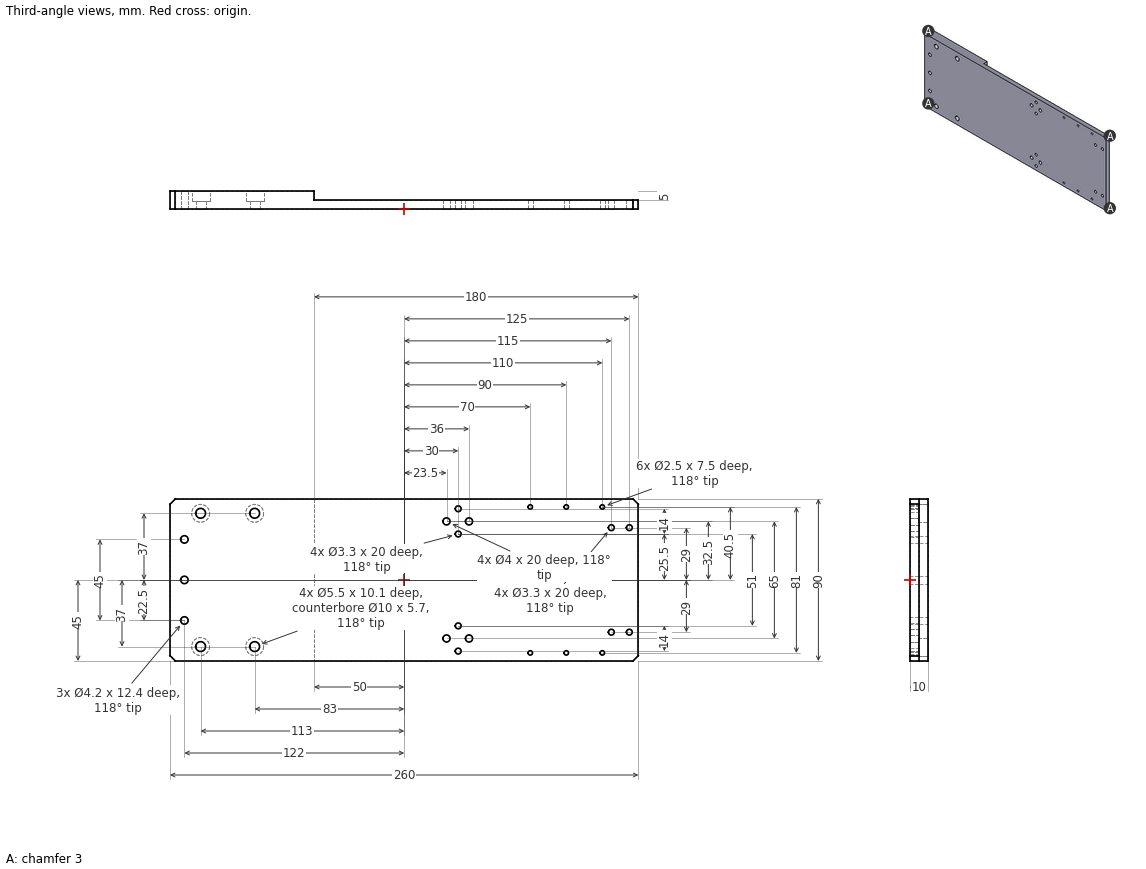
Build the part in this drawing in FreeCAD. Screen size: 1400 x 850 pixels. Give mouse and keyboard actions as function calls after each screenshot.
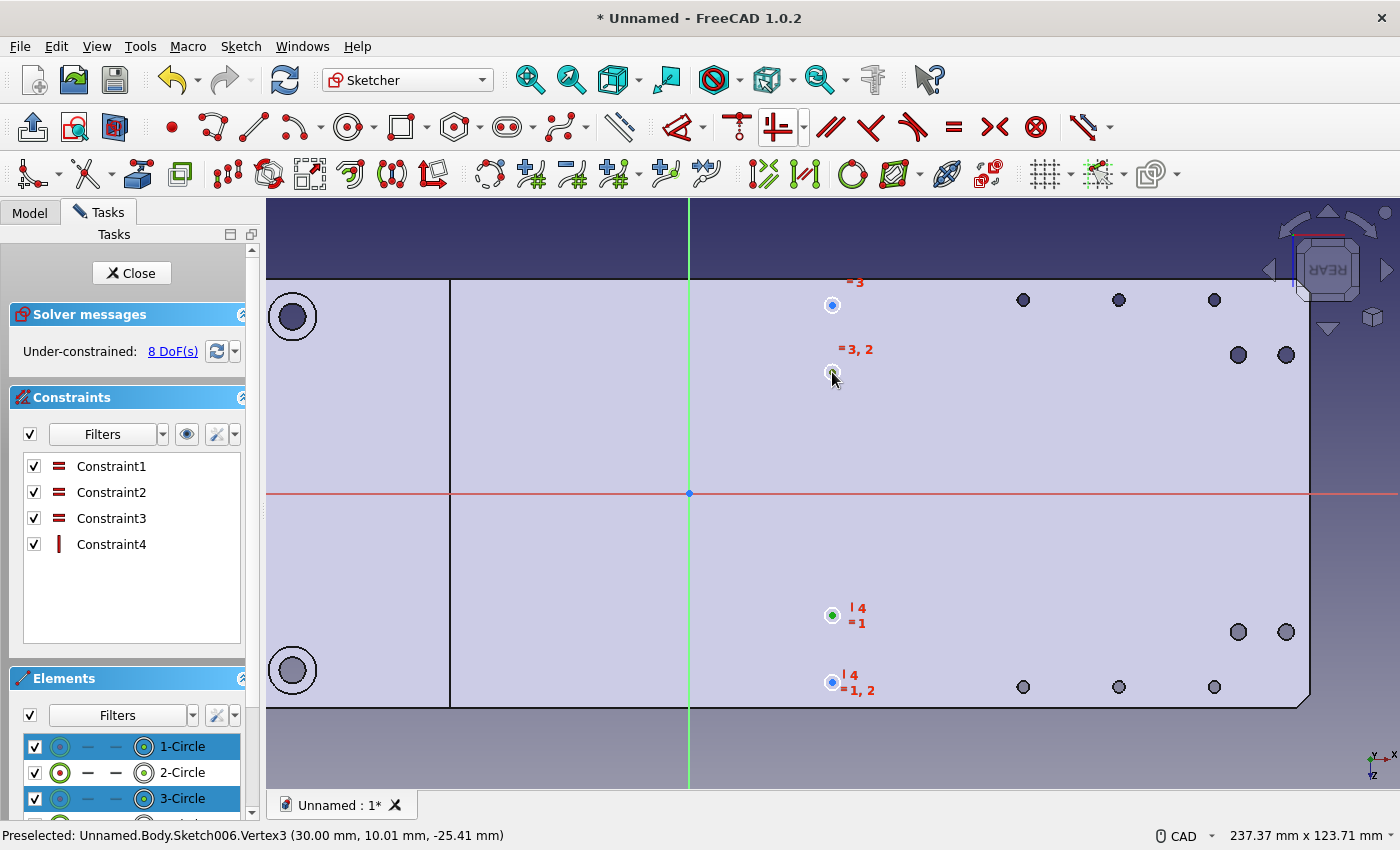
click(804, 128)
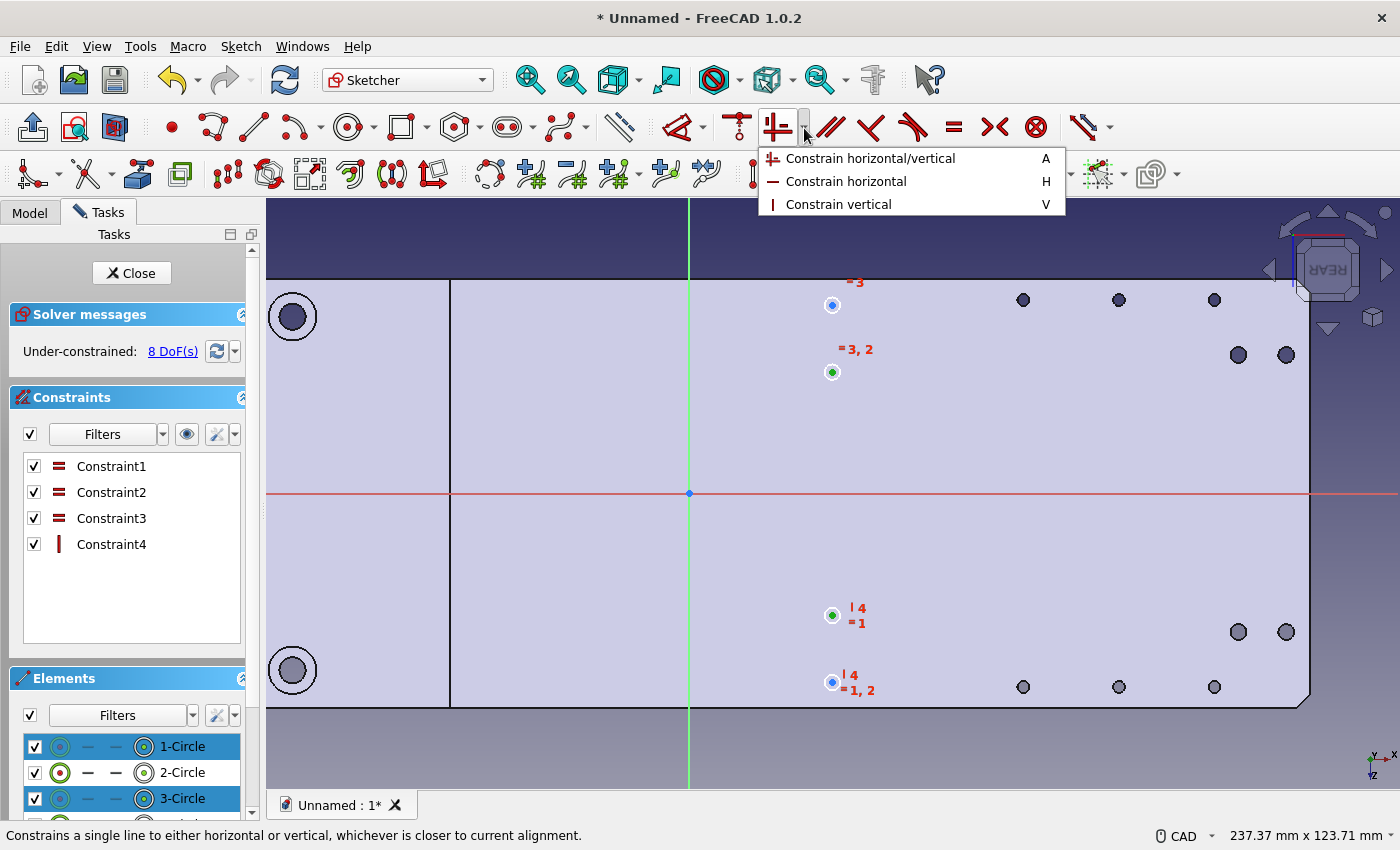
click(912, 204)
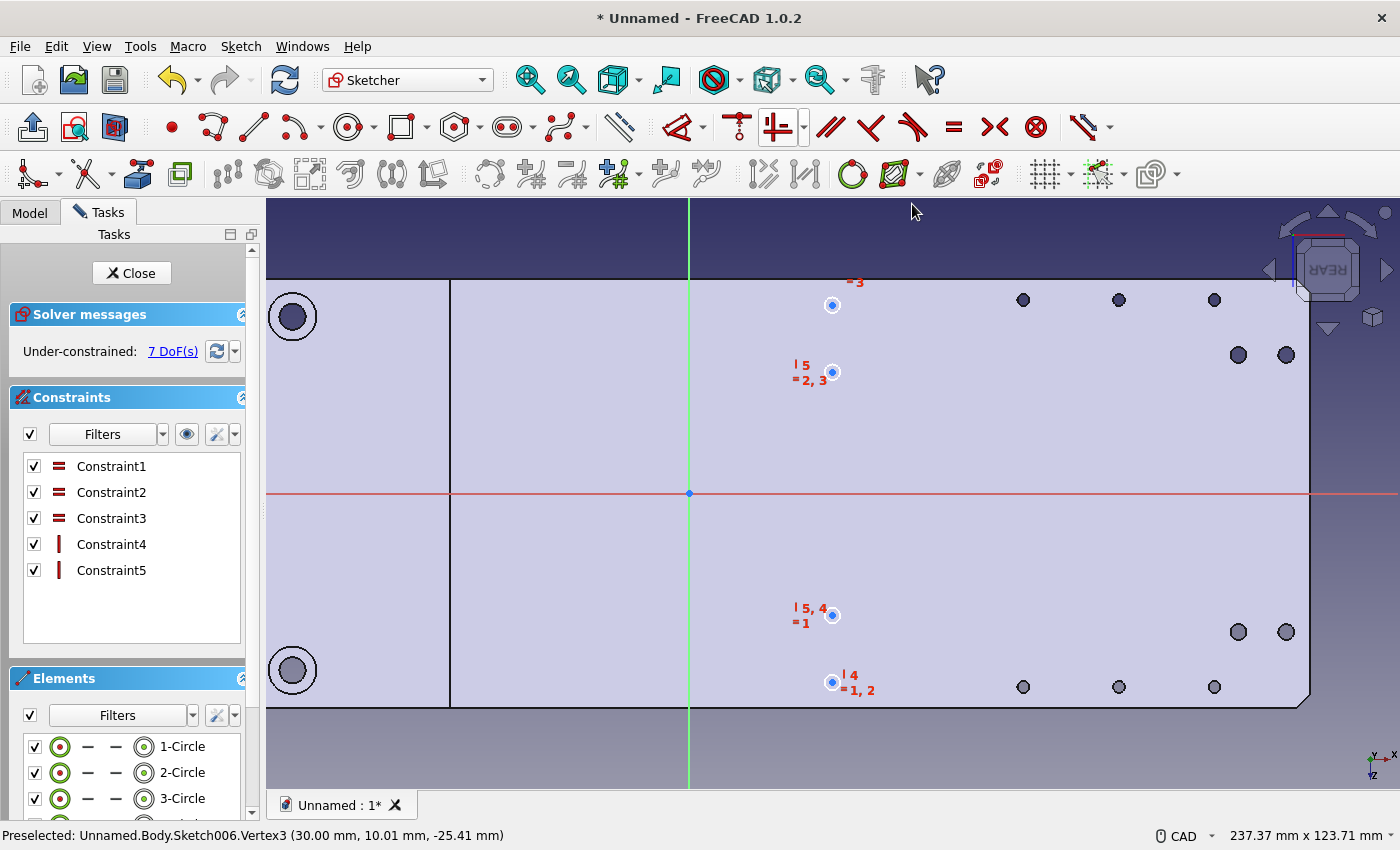
click(832, 372)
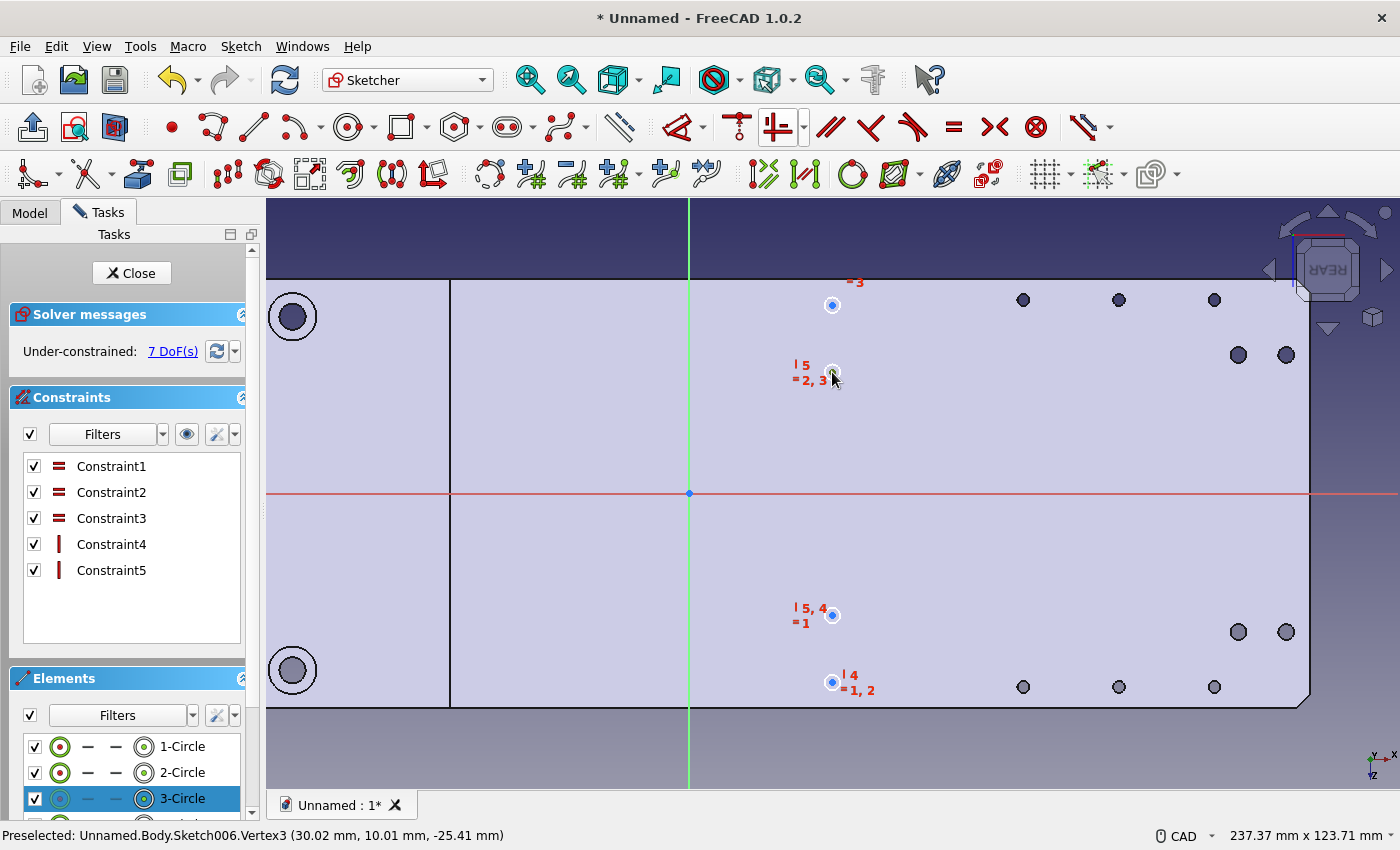
click(832, 305)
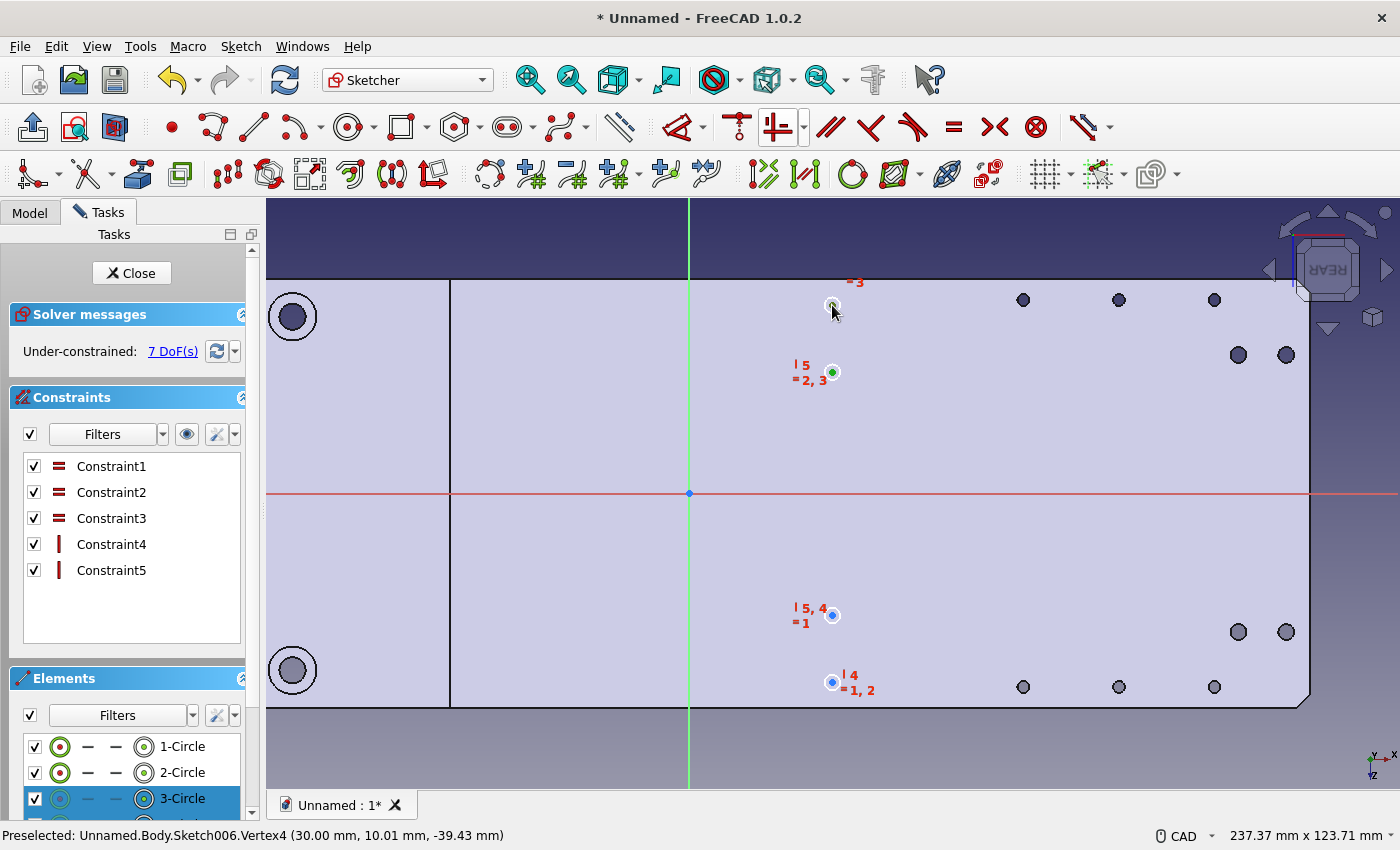
key(v)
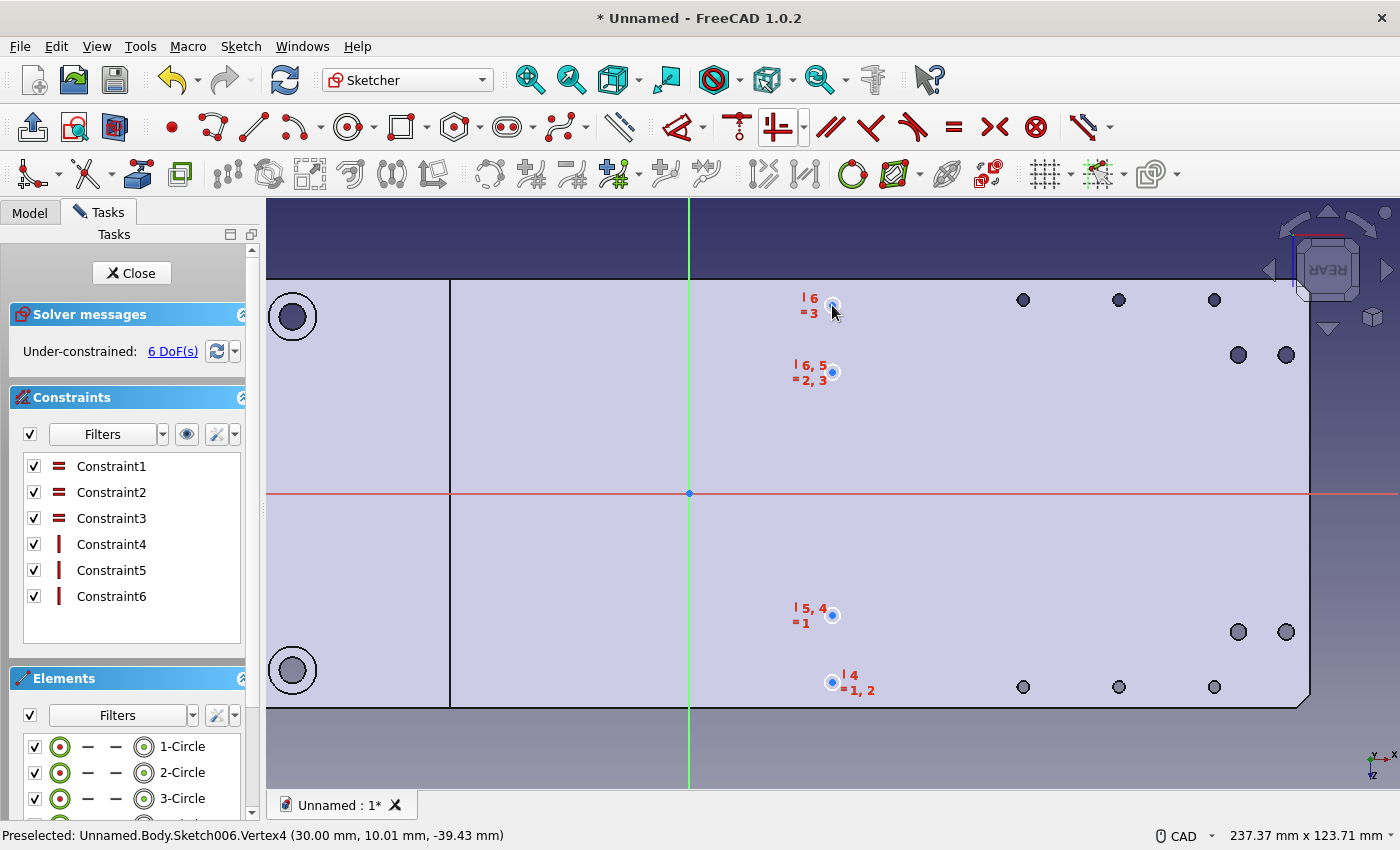
click(676, 128)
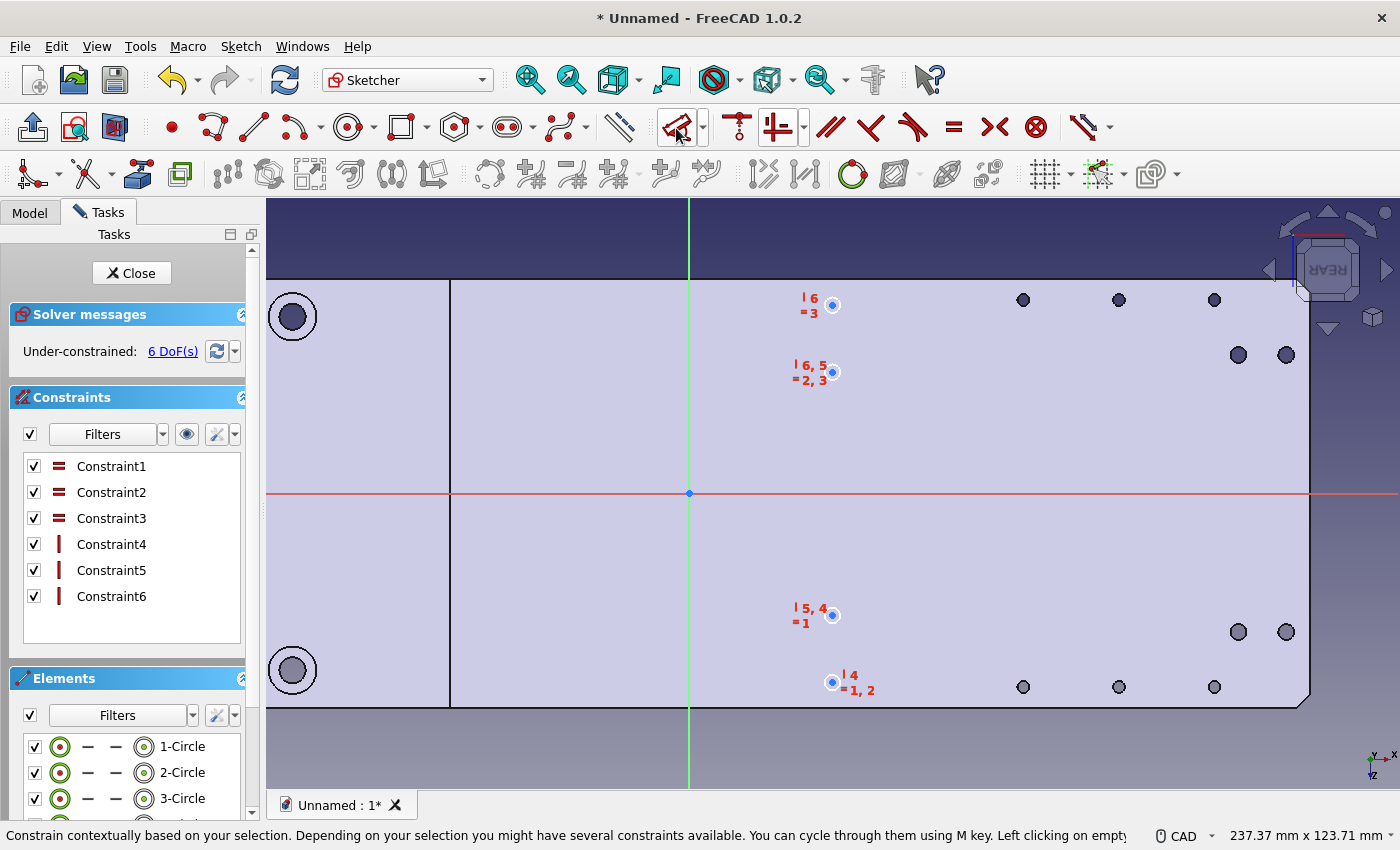
scroll(838, 610, up, 5)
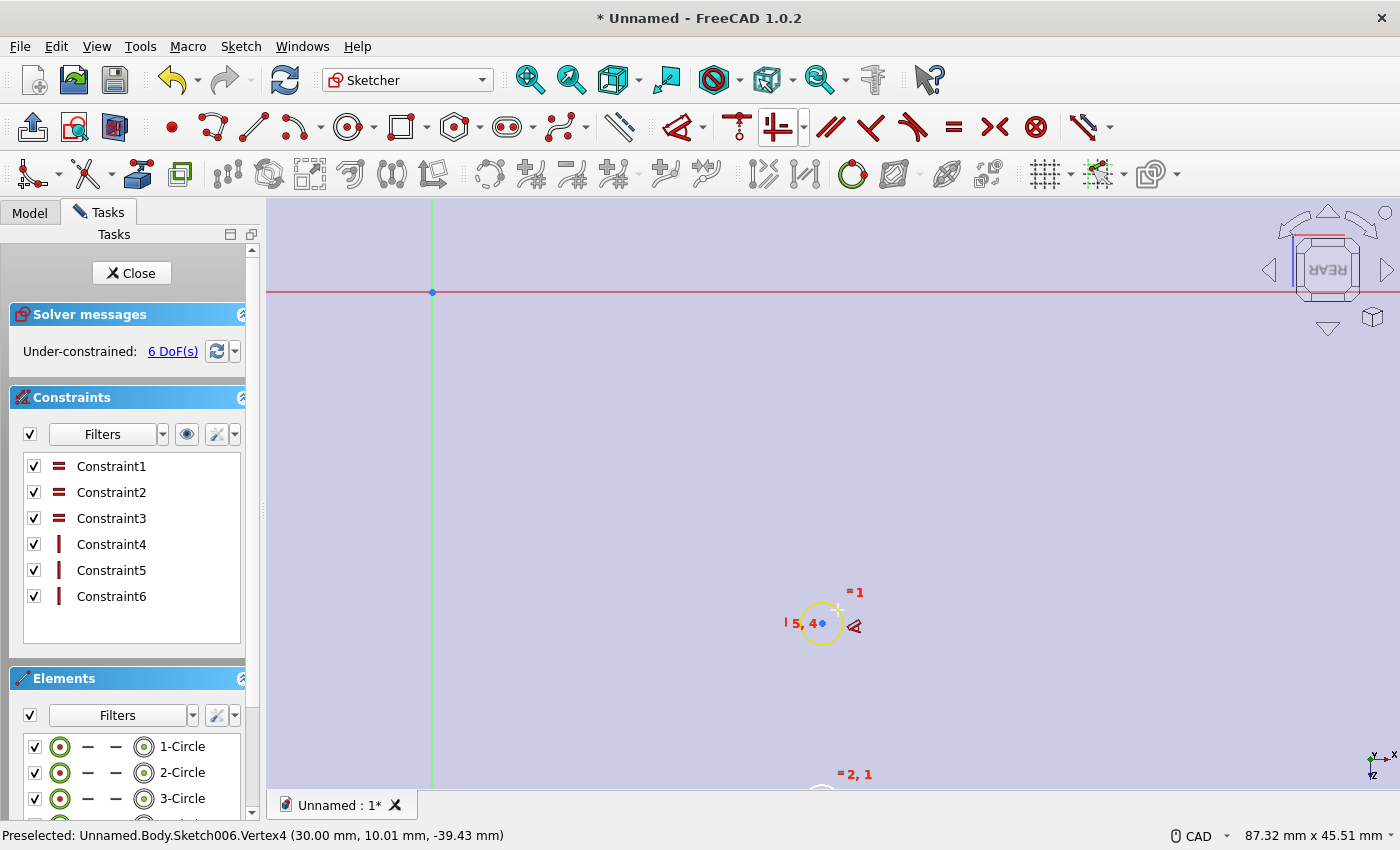
click(837, 609)
click(860, 587)